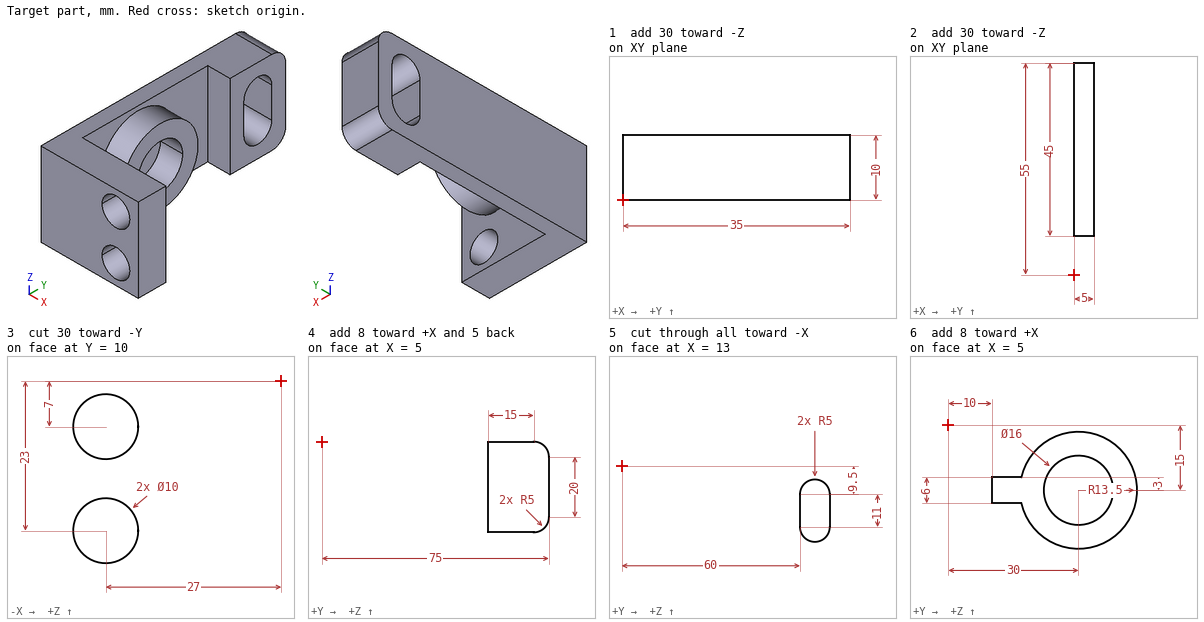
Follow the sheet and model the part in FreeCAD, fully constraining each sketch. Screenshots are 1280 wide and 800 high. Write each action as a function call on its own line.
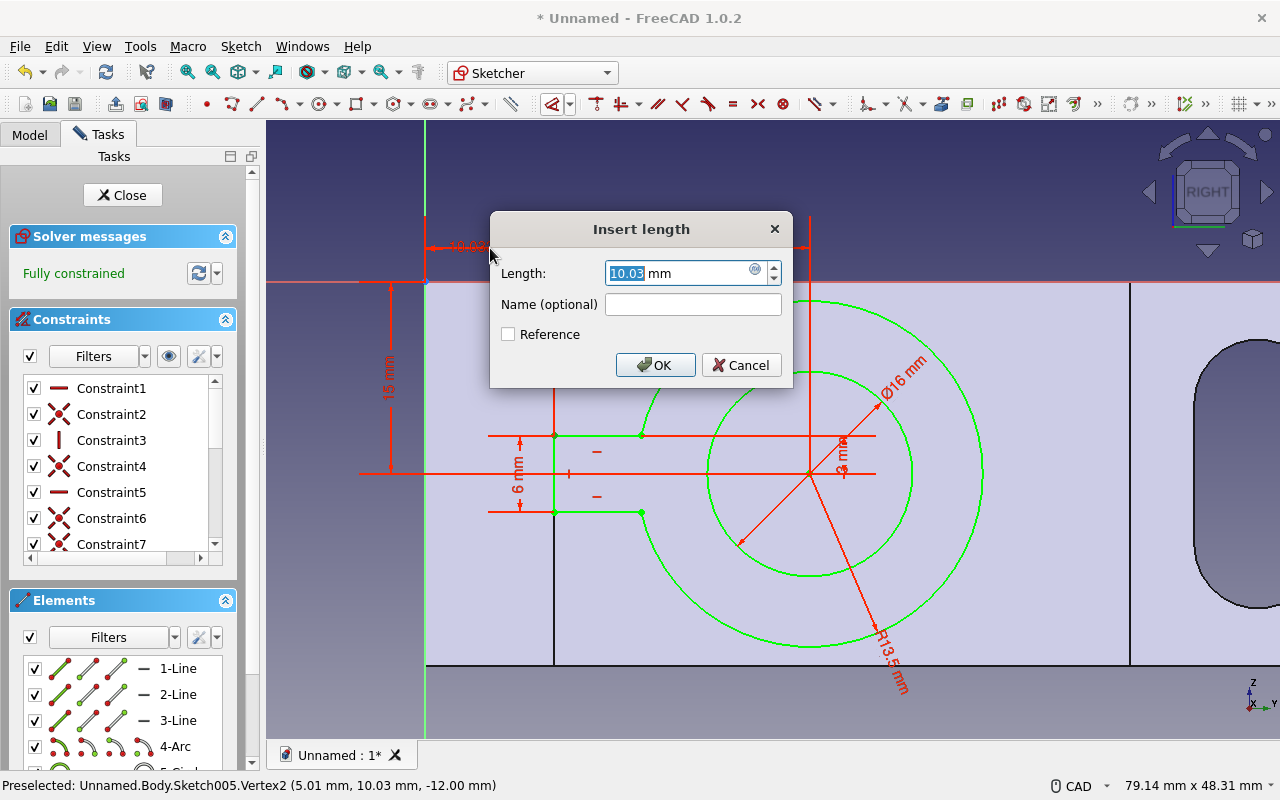
text(10)
key(Return)
key(Escape)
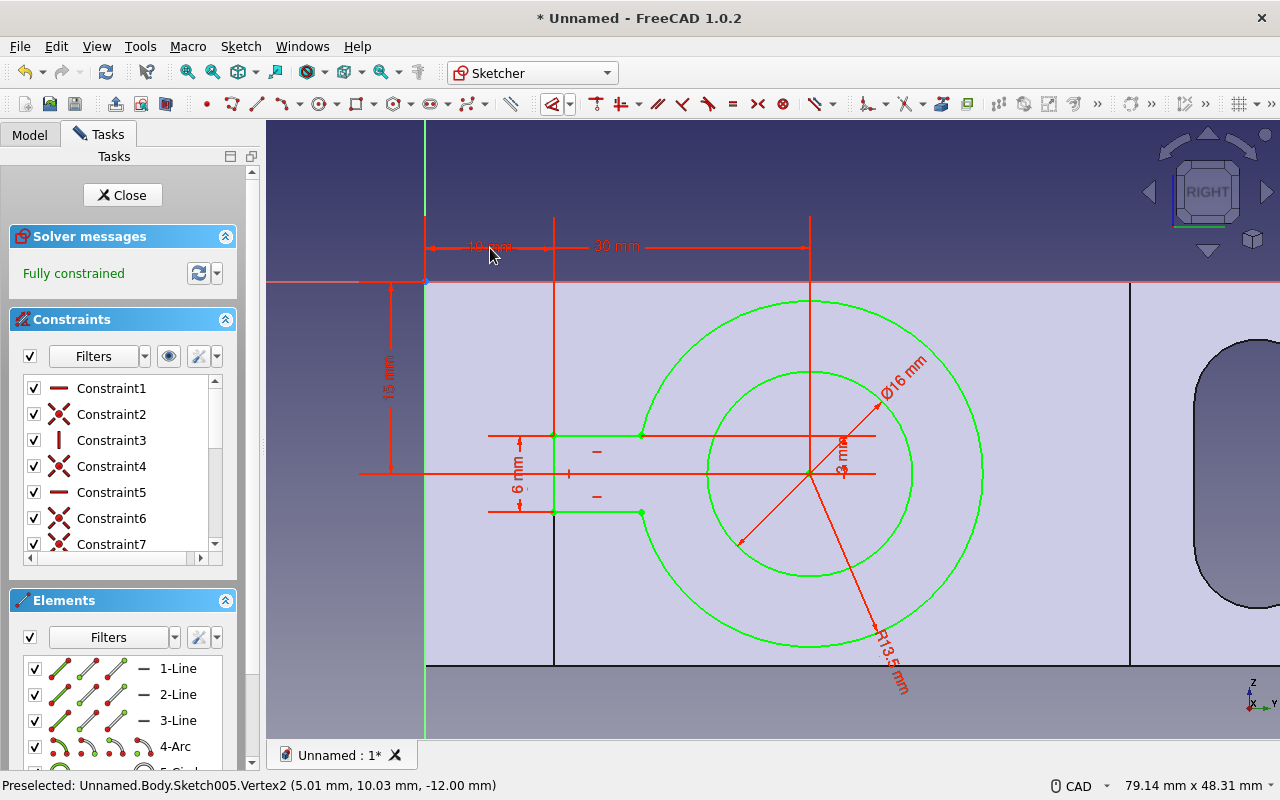
click(123, 195)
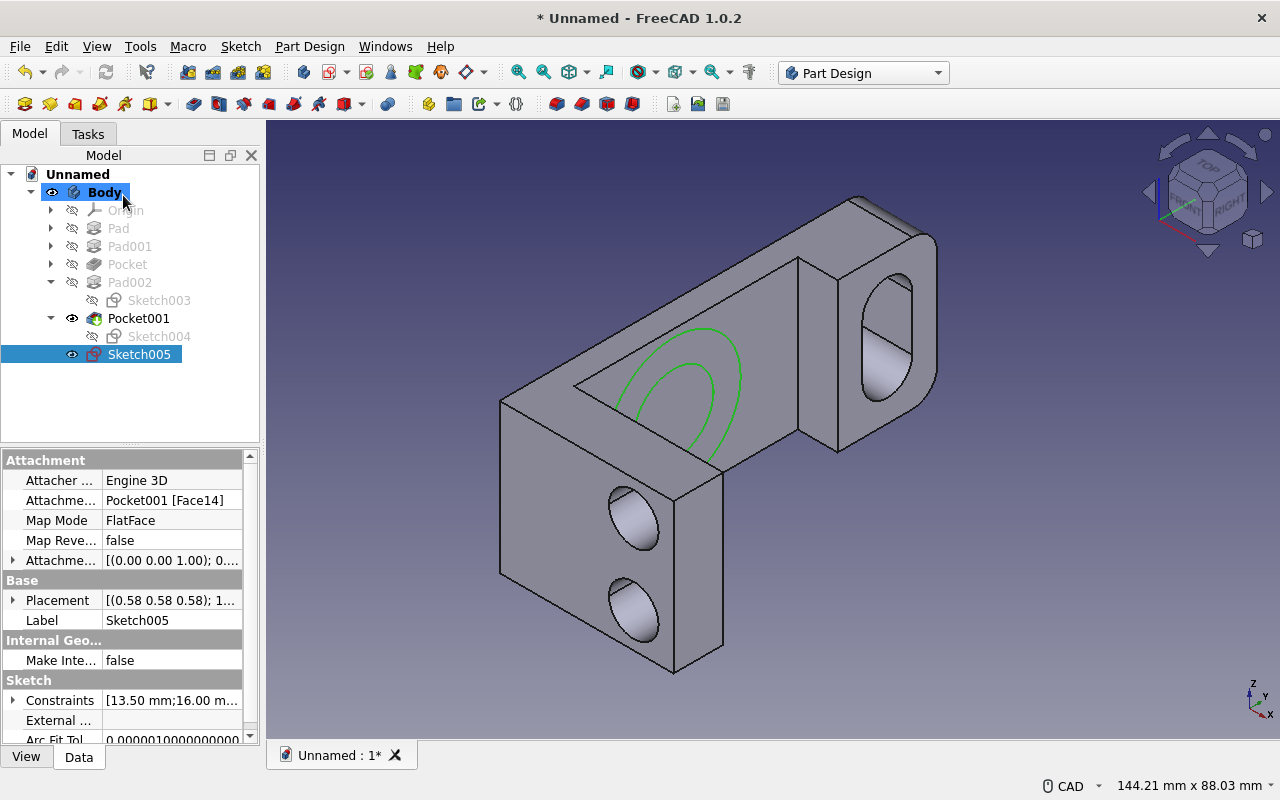
click(25, 104)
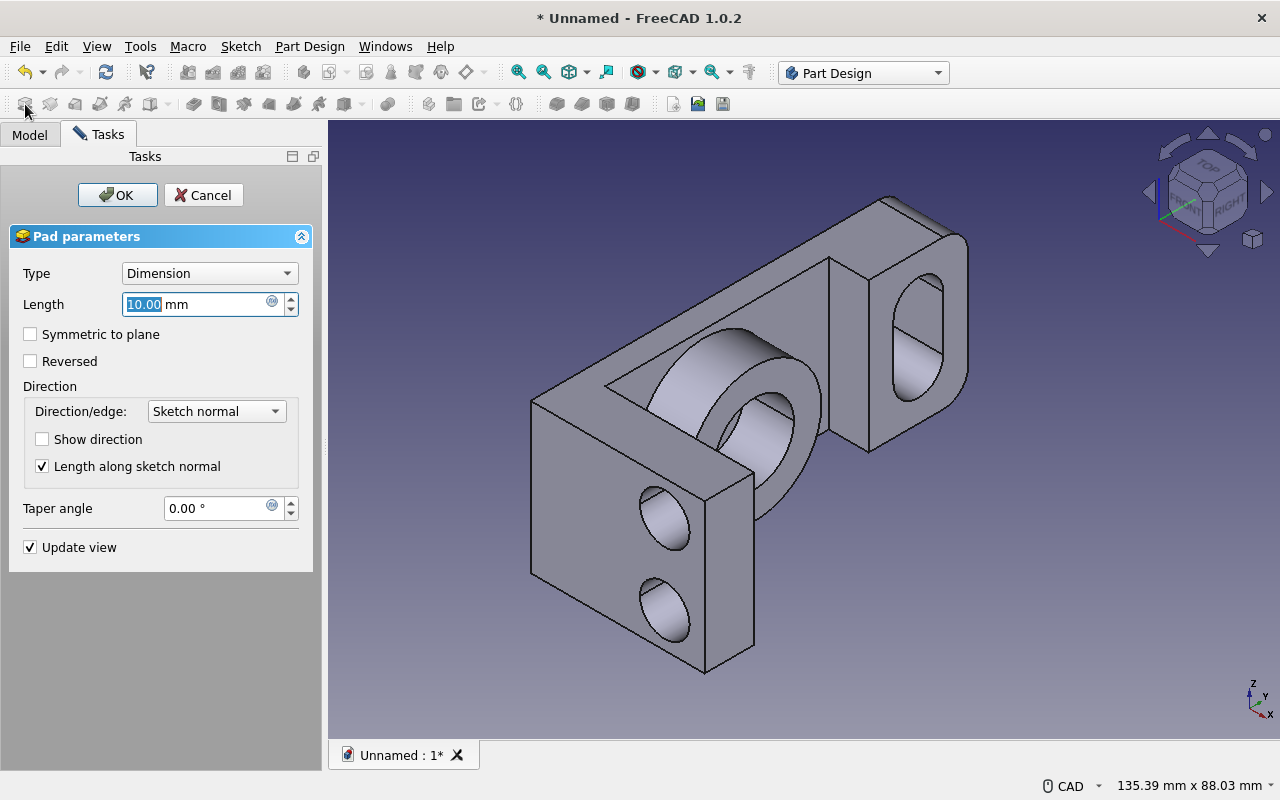
text(8)
key(Tab)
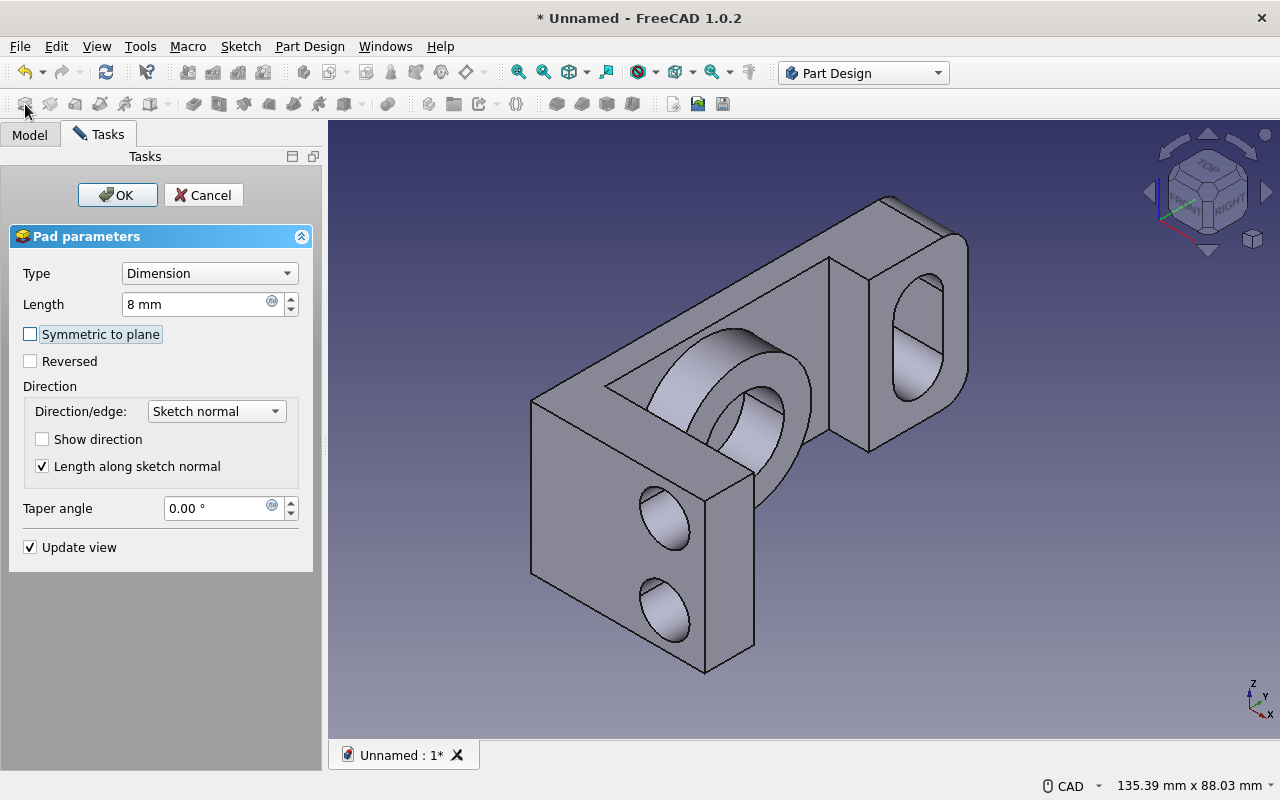
click(118, 195)